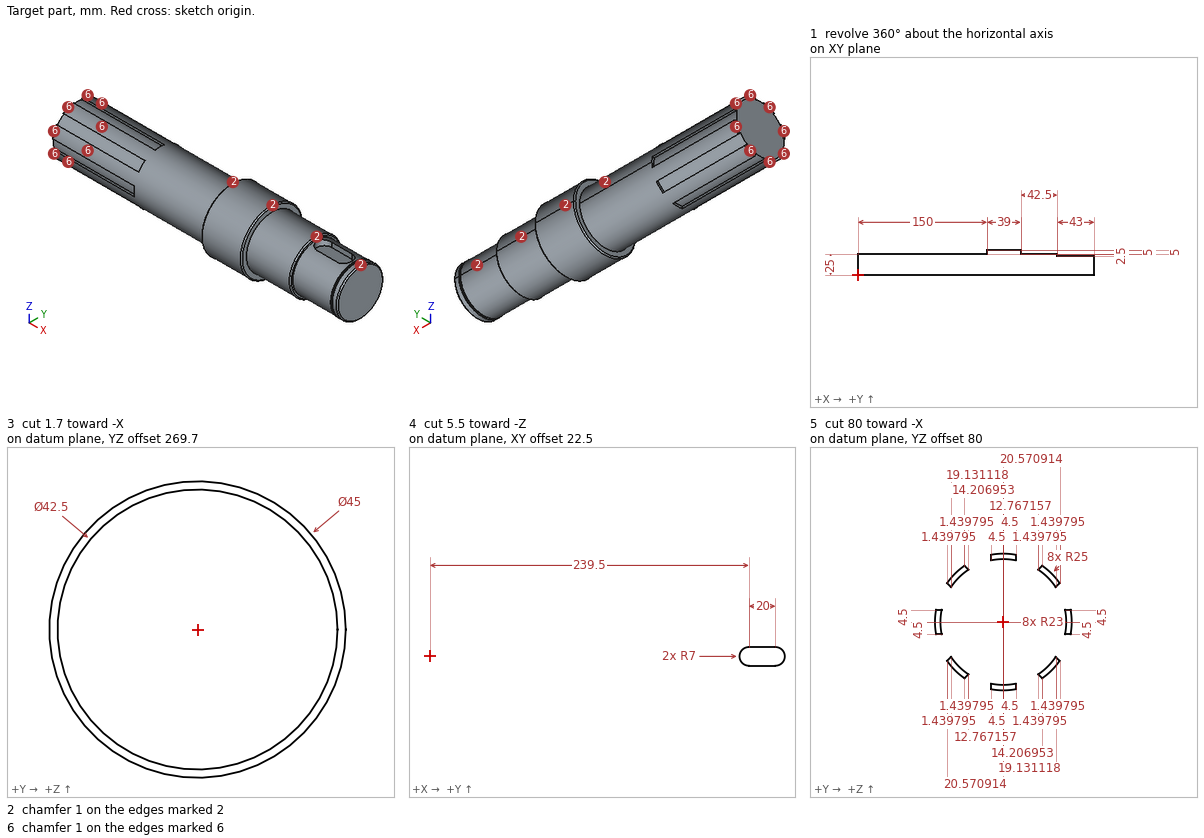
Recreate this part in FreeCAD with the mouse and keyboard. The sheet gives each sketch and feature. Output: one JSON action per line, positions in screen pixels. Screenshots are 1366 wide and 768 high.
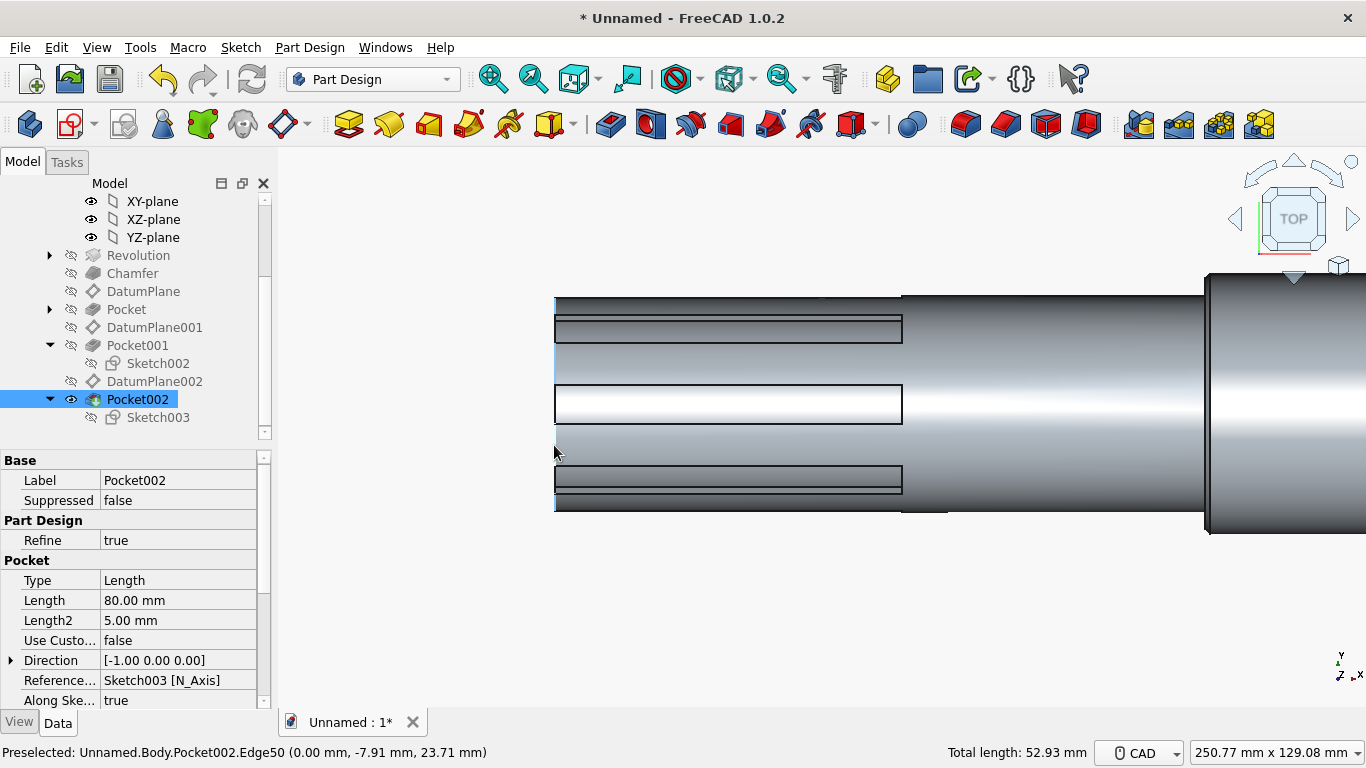
{"action": "left_click", "coordinate": [494, 80]}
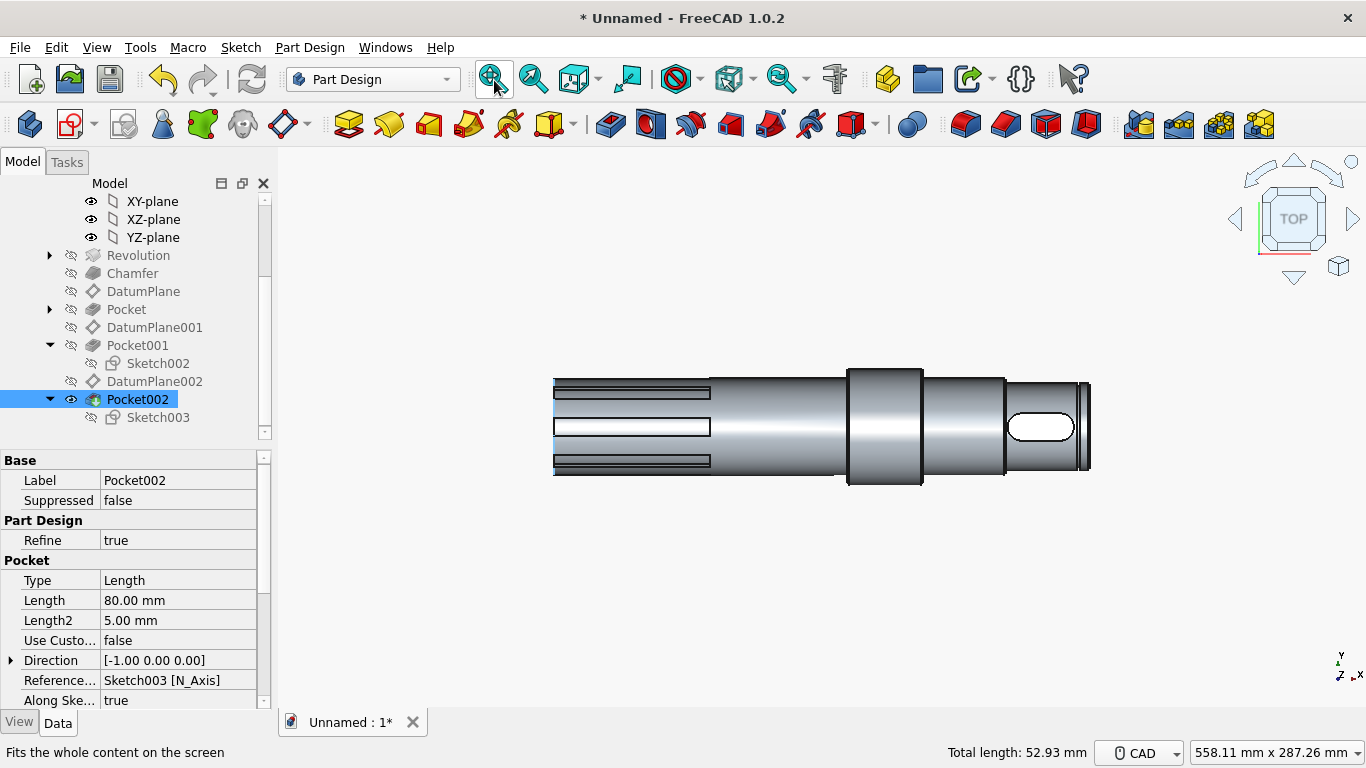
{"action": "key", "text": "1"}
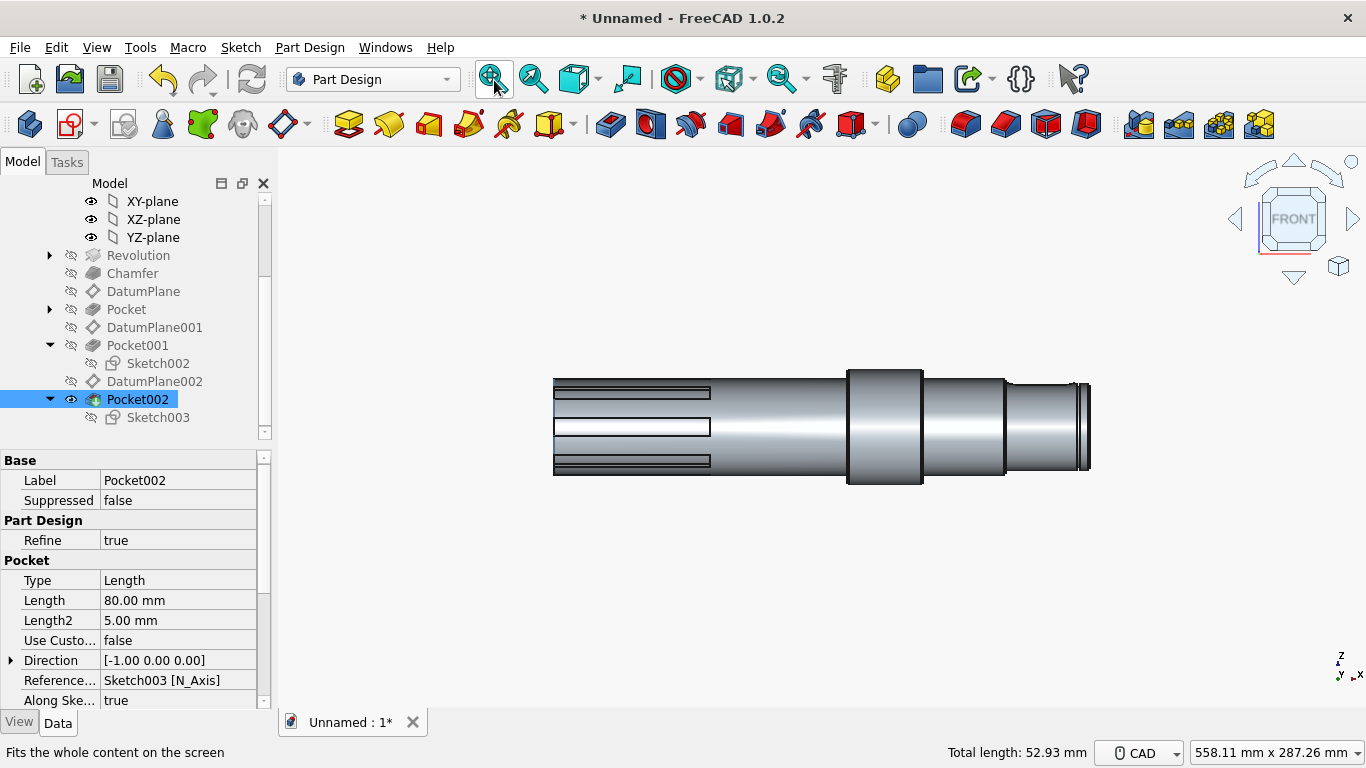
{"action": "left_click", "coordinate": [554, 473], "text": "ctrl"}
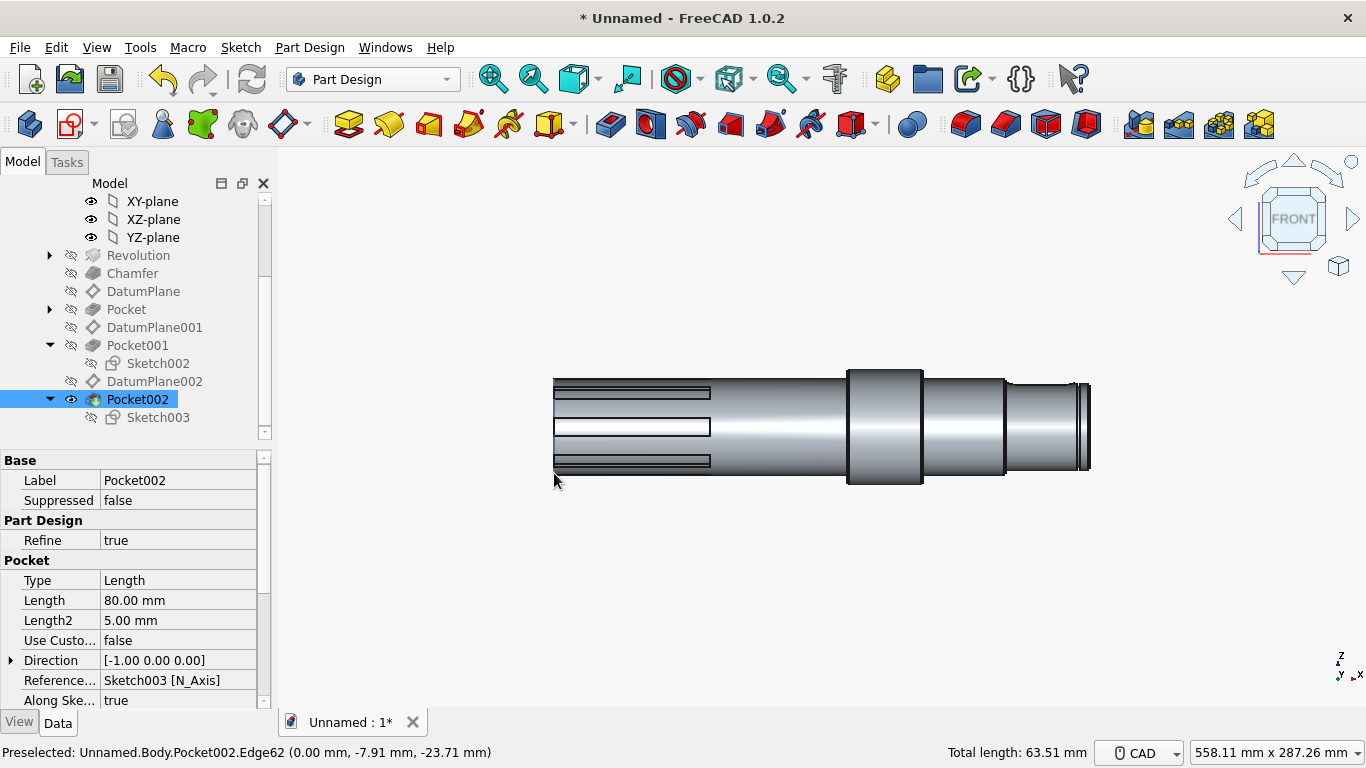
{"action": "scroll", "coordinate": [554, 471], "scroll_direction": "up", "scroll_amount": 4}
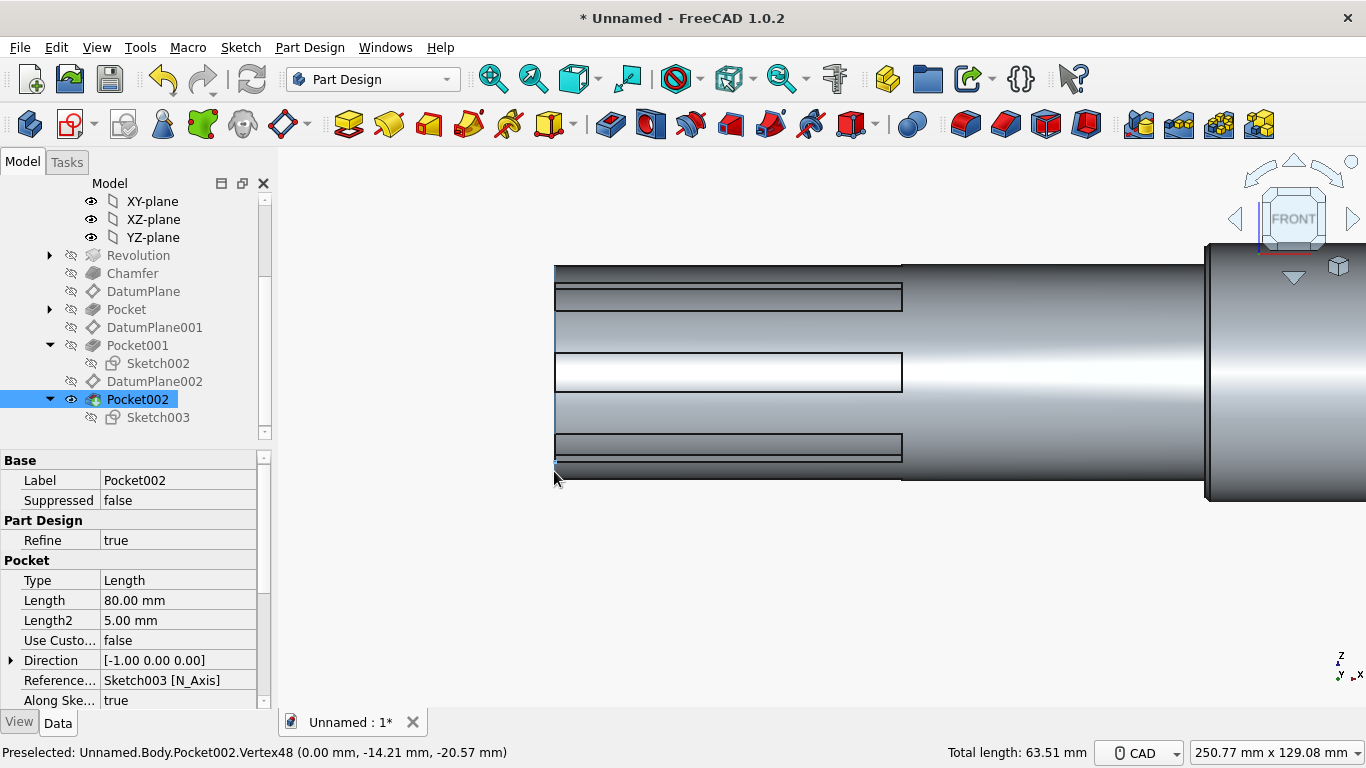
{"action": "left_click", "coordinate": [494, 80]}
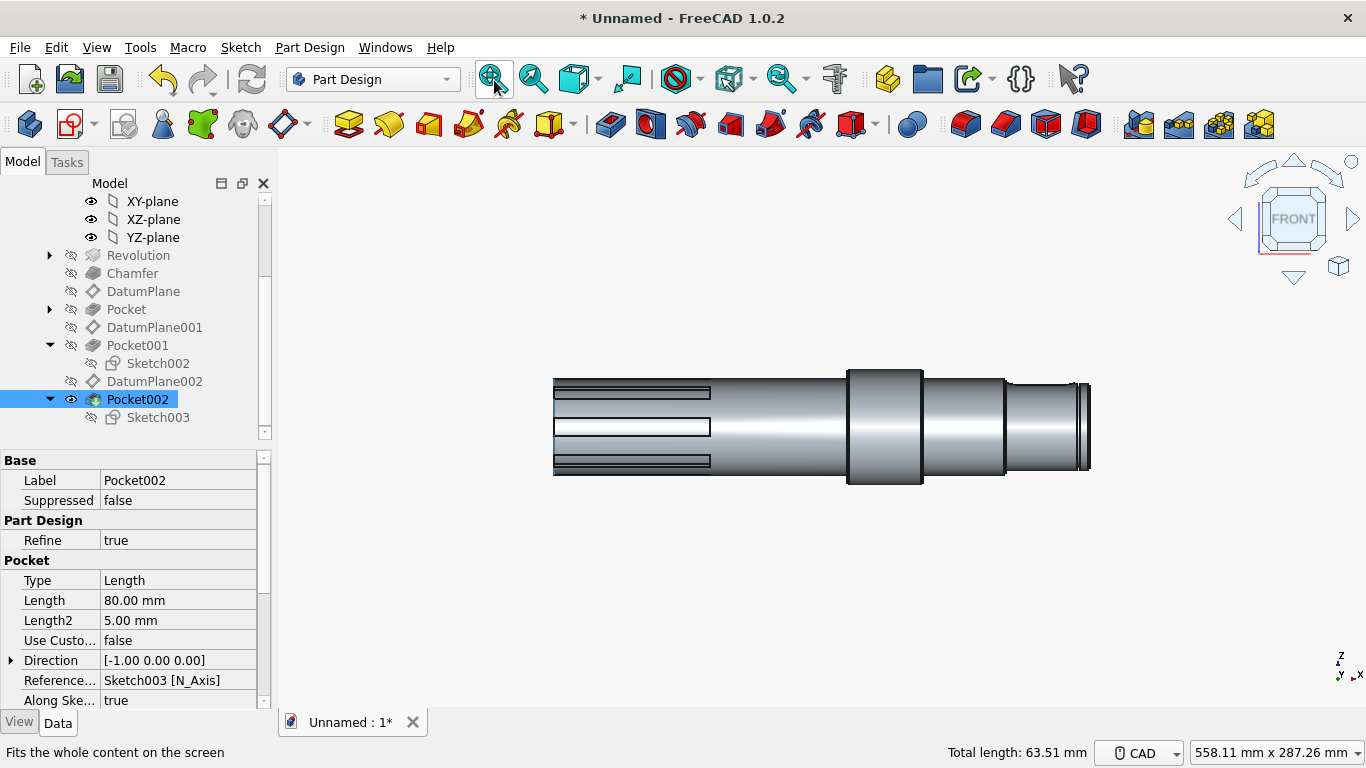
{"action": "key", "text": "3"}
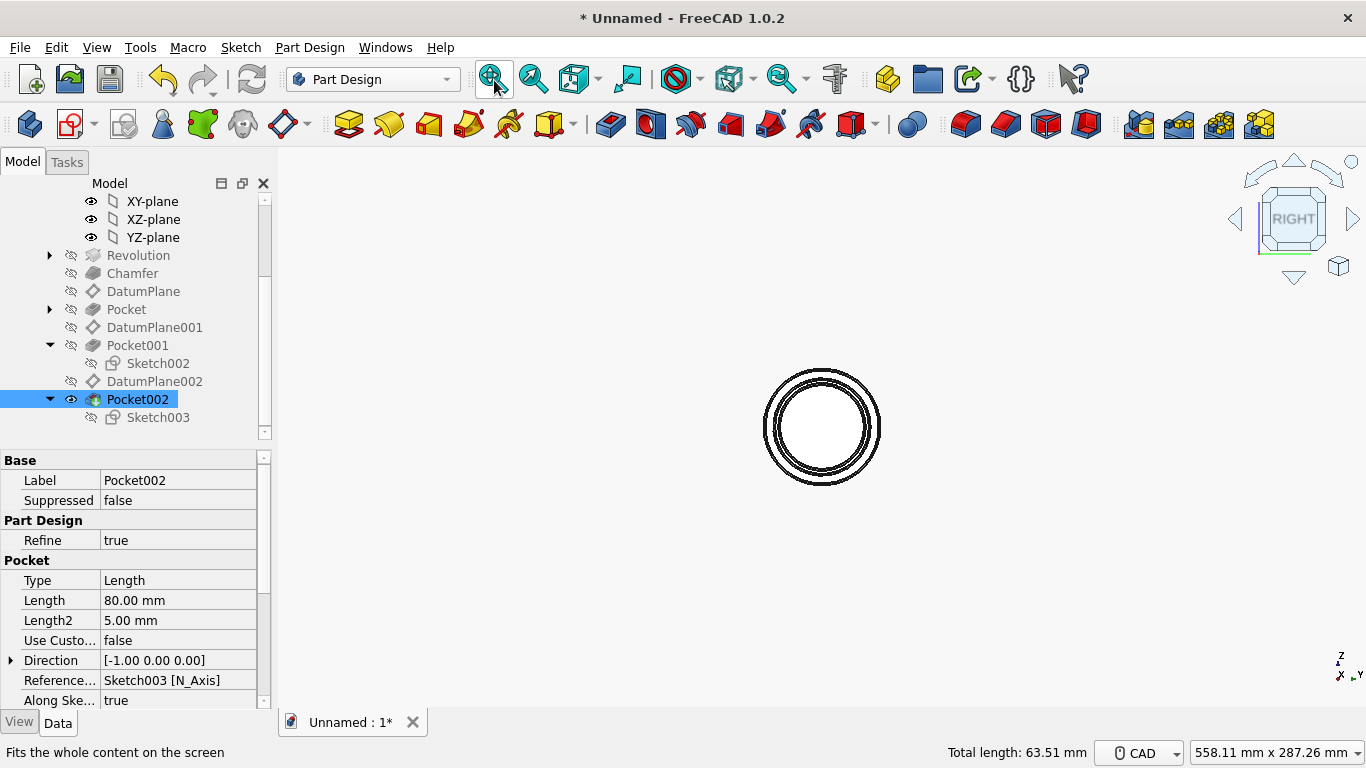
{"action": "left_click", "coordinate": [494, 80]}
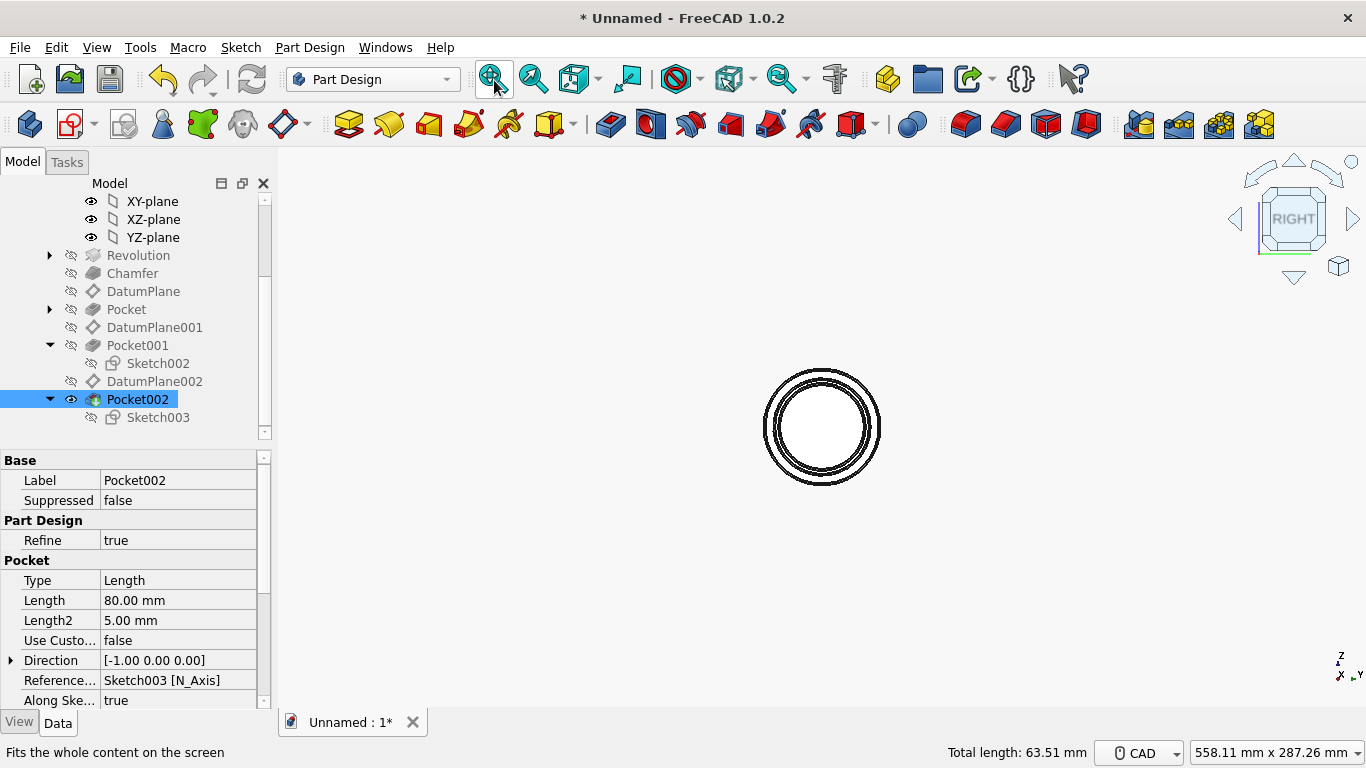
{"action": "scroll", "coordinate": [841, 471], "scroll_direction": "up", "scroll_amount": 4}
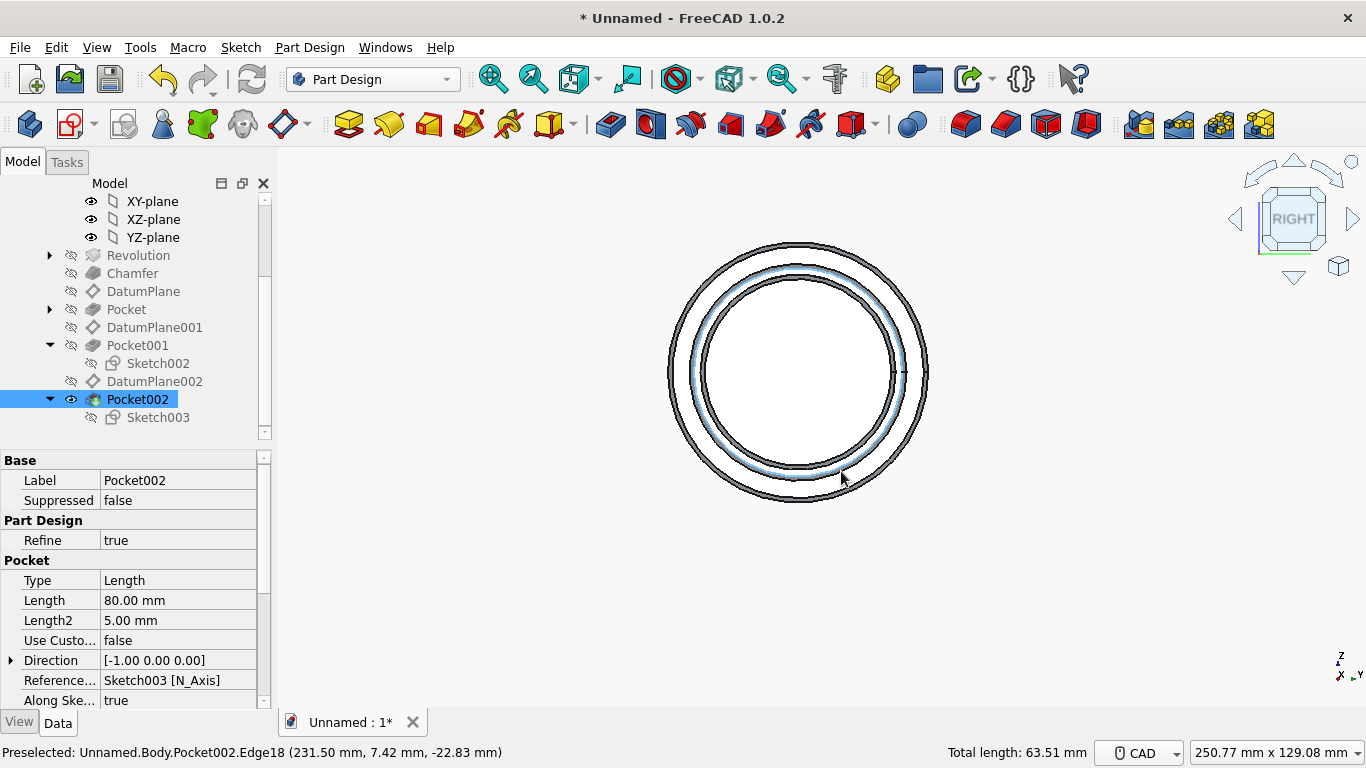
{"action": "key", "text": "v f"}